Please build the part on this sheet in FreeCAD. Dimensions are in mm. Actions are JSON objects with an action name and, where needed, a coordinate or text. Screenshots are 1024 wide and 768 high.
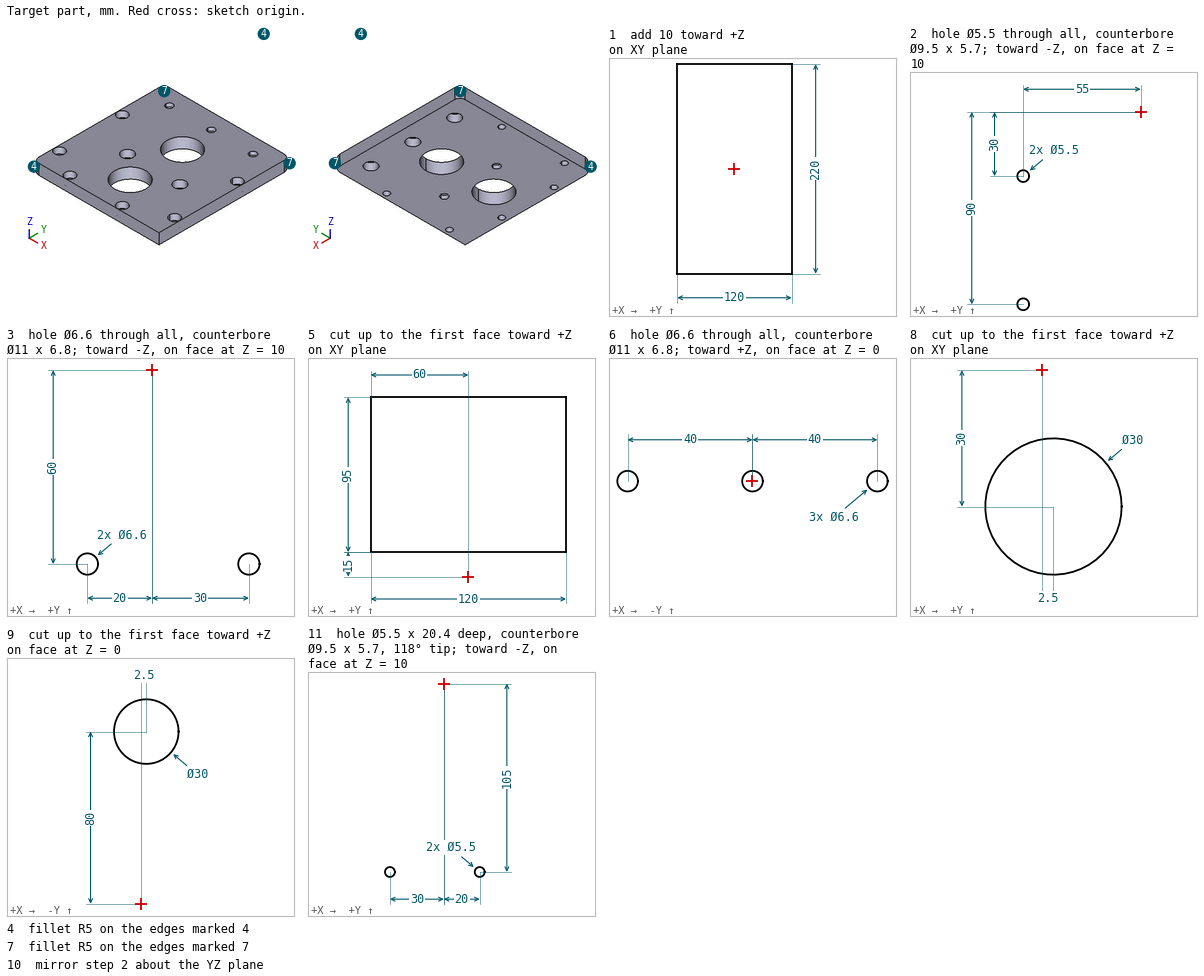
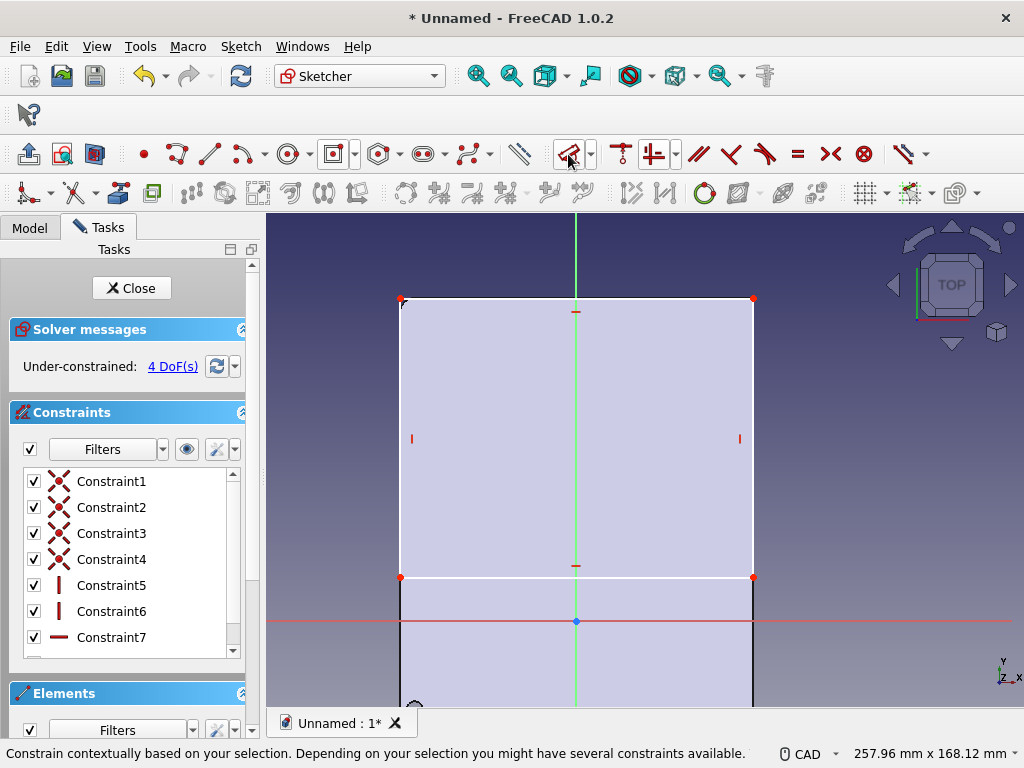
{"action": "left_click", "coordinate": [400, 383]}
{"action": "left_click", "coordinate": [366, 438]}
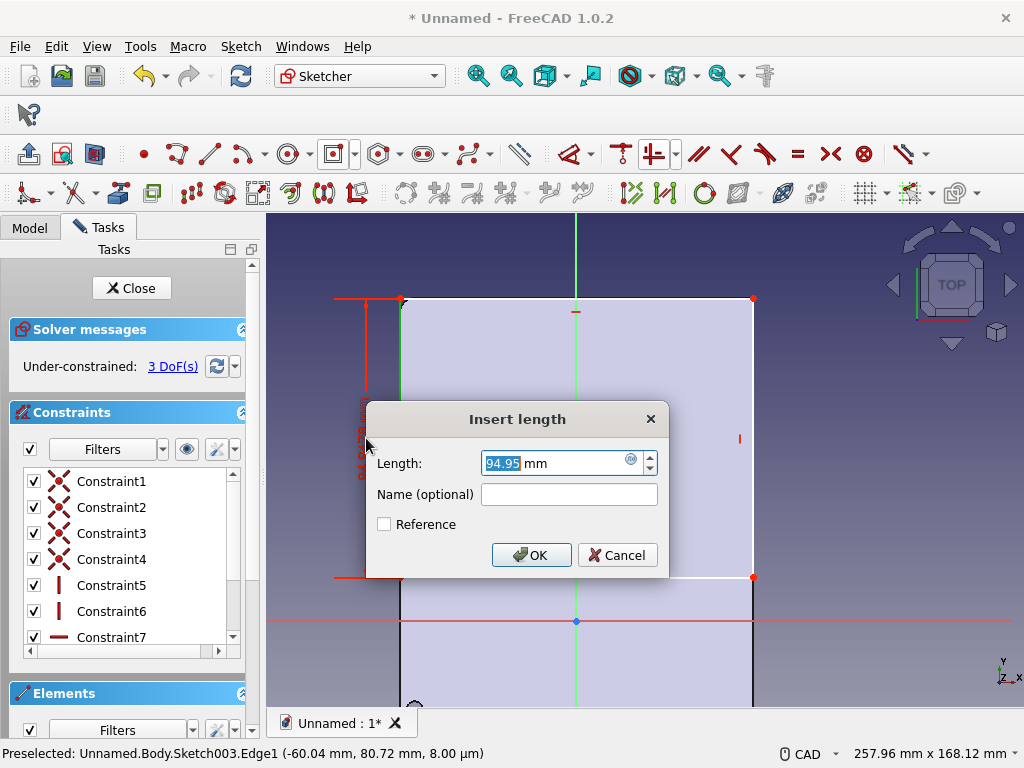
{"action": "type", "text": "95"}
{"action": "key", "text": "Return"}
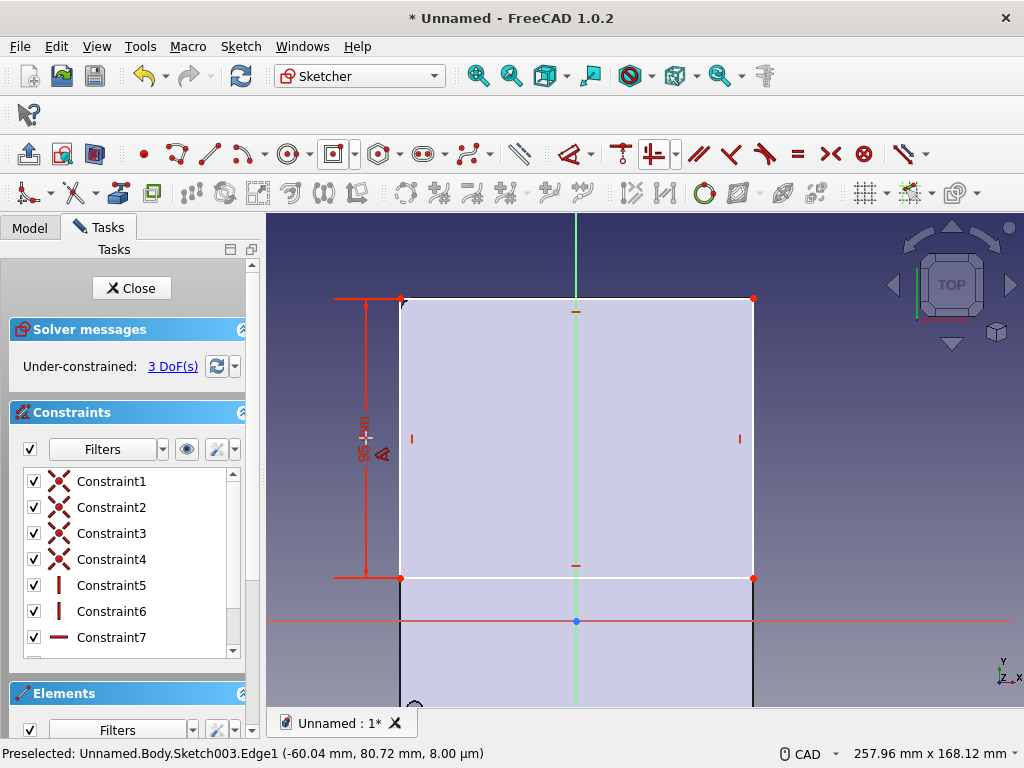
{"action": "left_click", "coordinate": [506, 578]}
{"action": "left_click", "coordinate": [495, 544]}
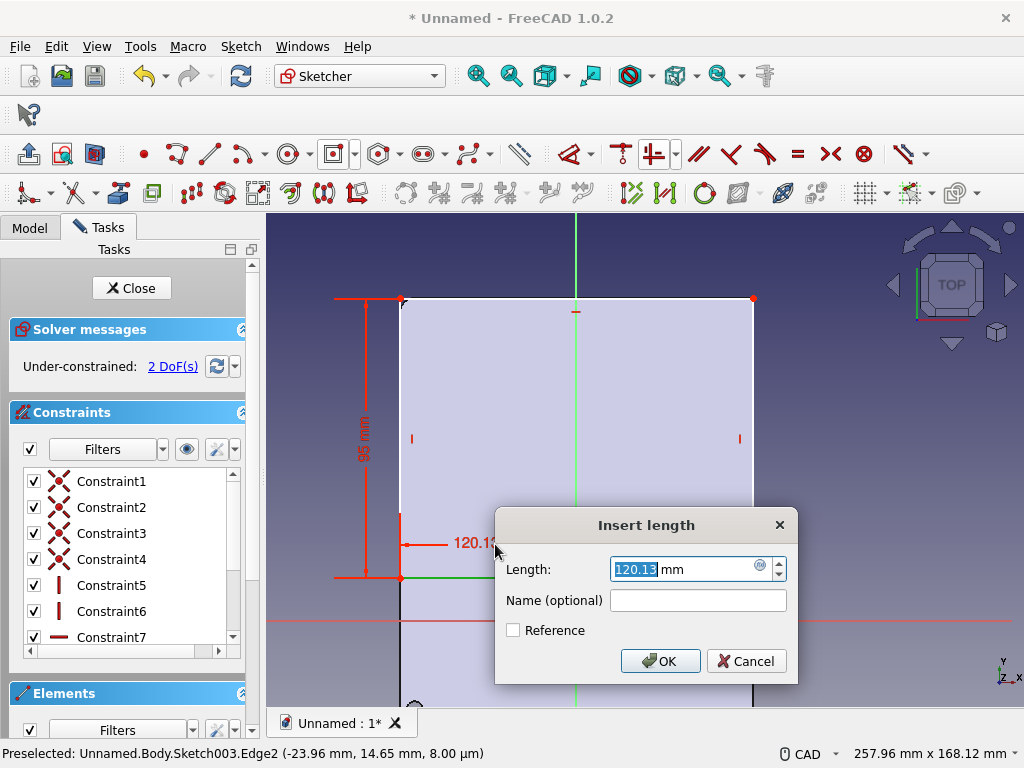
{"action": "type", "text": "120"}
{"action": "key", "text": "Return"}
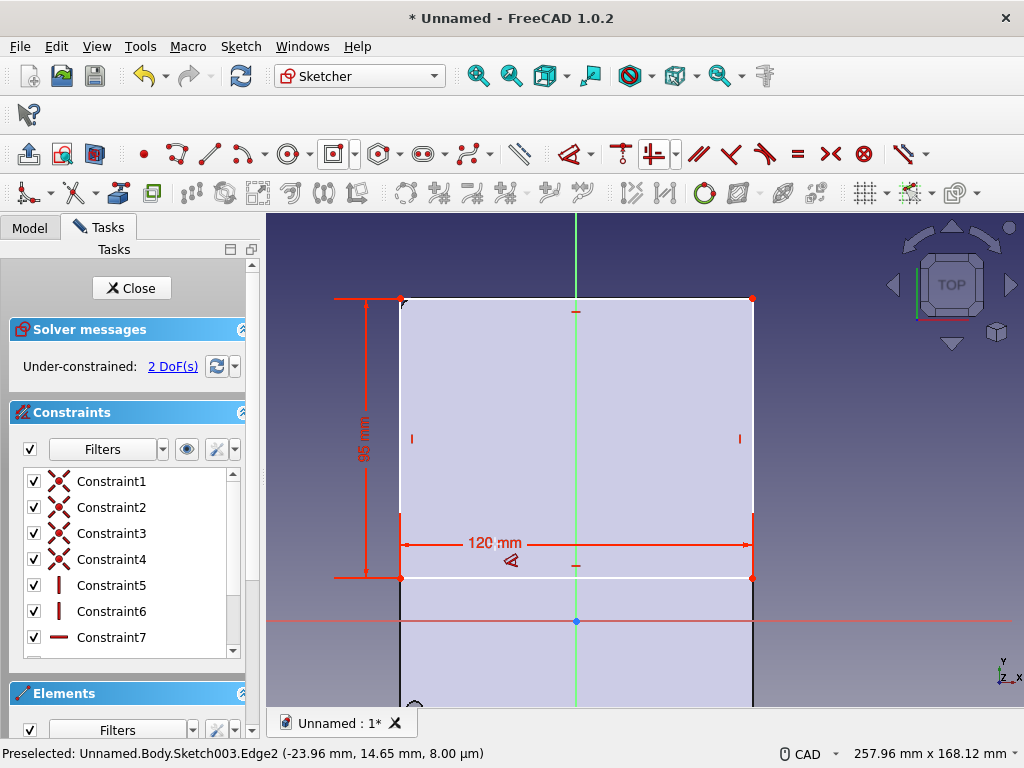
{"action": "left_click", "coordinate": [400, 299]}
{"action": "left_click", "coordinate": [488, 655]}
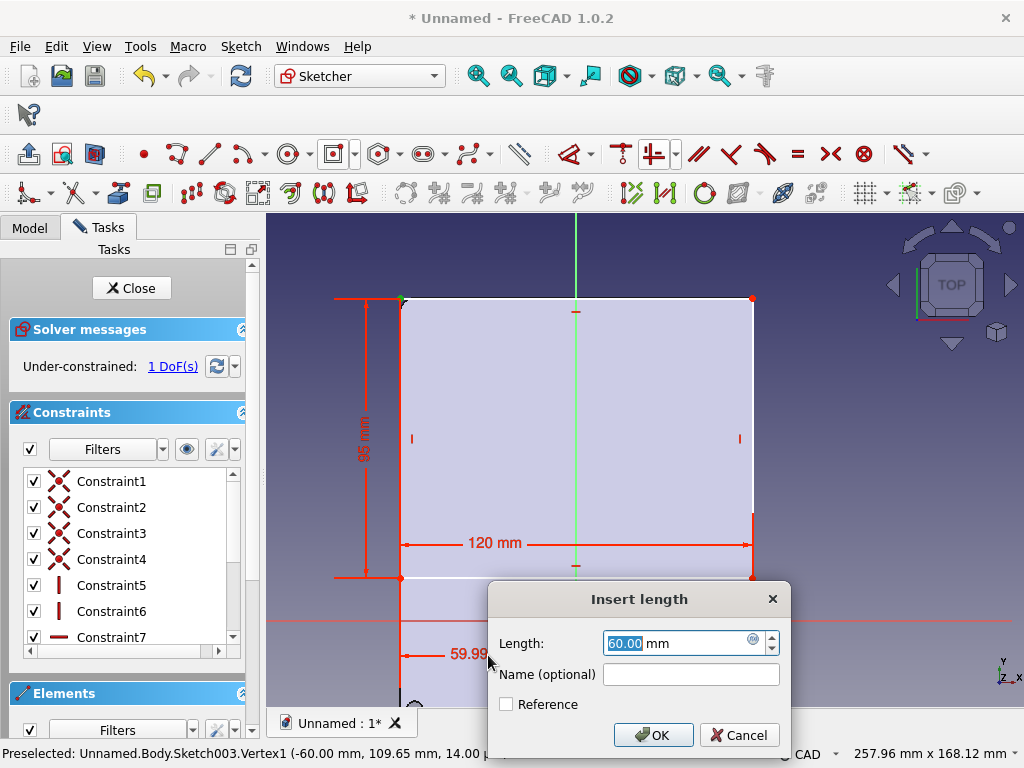
{"action": "type", "text": "60"}
{"action": "key", "text": "Return"}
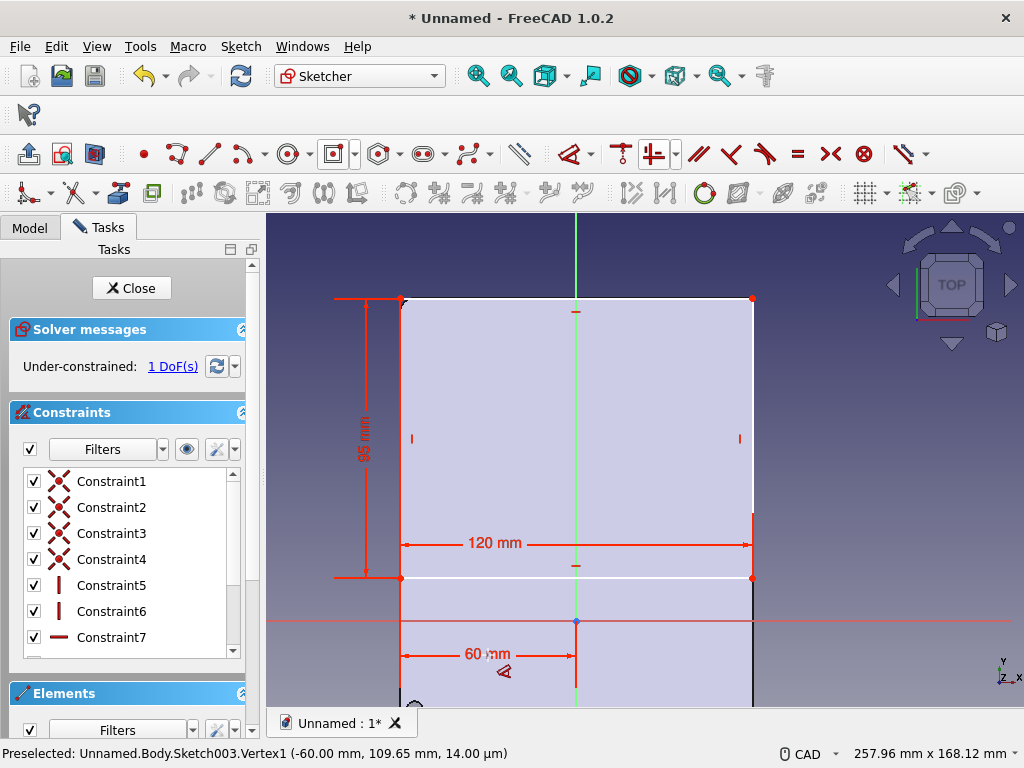
{"action": "left_click", "coordinate": [400, 578]}
{"action": "left_click", "coordinate": [366, 600]}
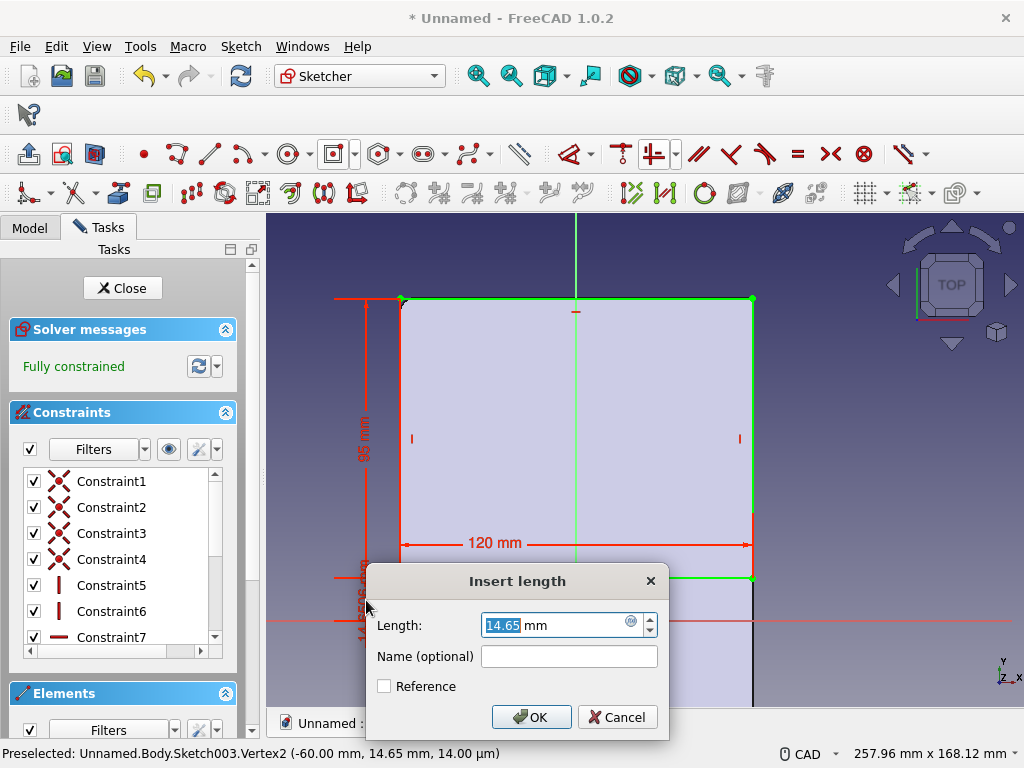
{"action": "type", "text": "15"}
{"action": "key", "text": "Return"}
{"action": "key", "text": "Escape"}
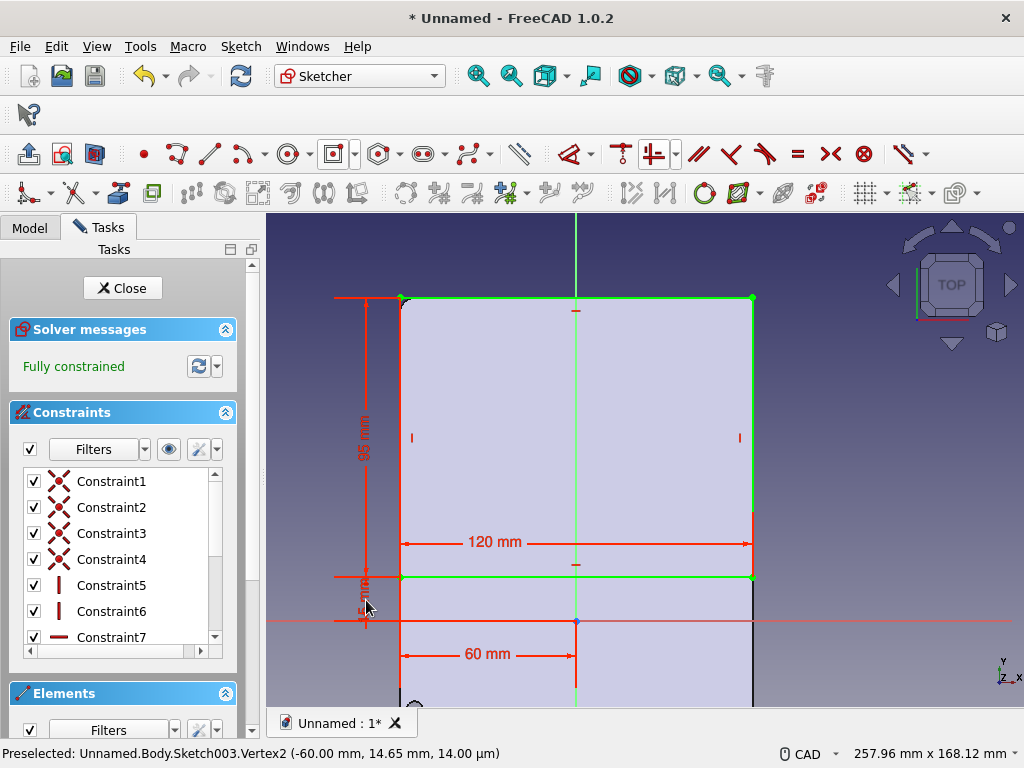
{"action": "left_click", "coordinate": [123, 288]}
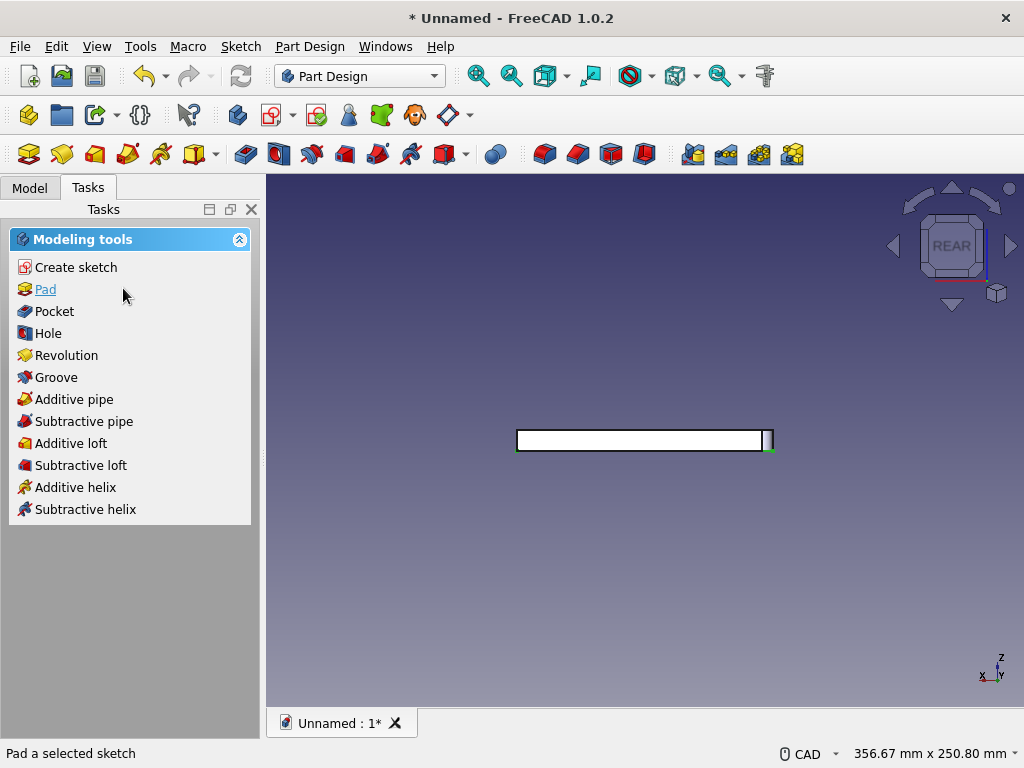
{"action": "left_click", "coordinate": [246, 154]}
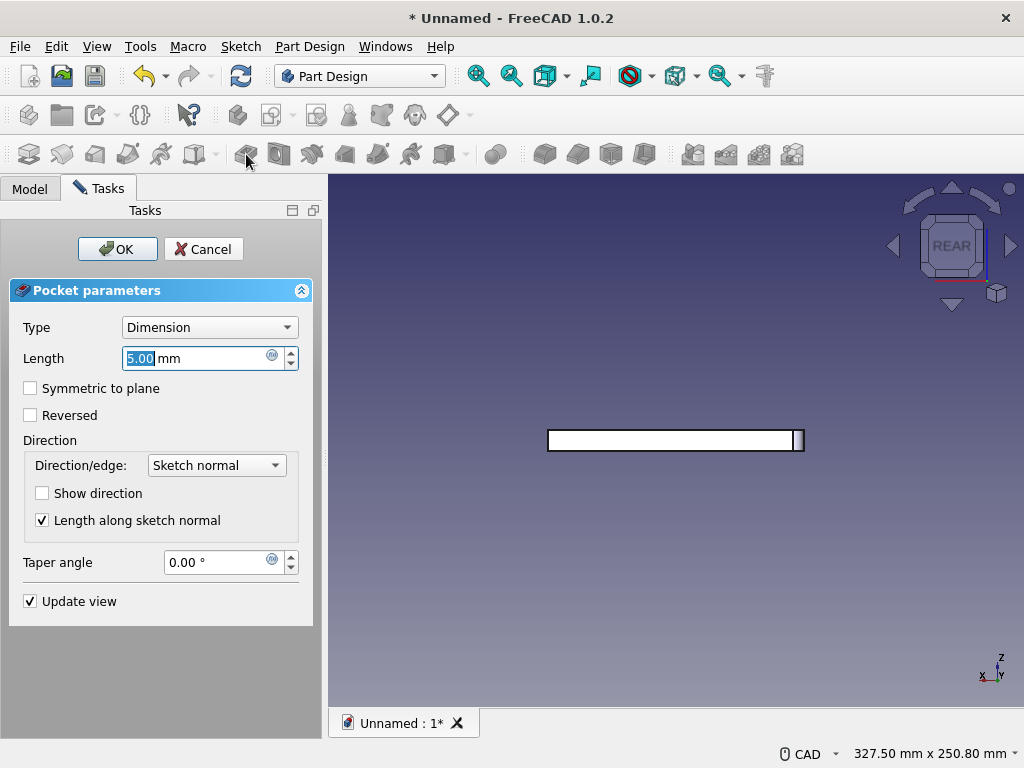
{"action": "left_click", "coordinate": [210, 328]}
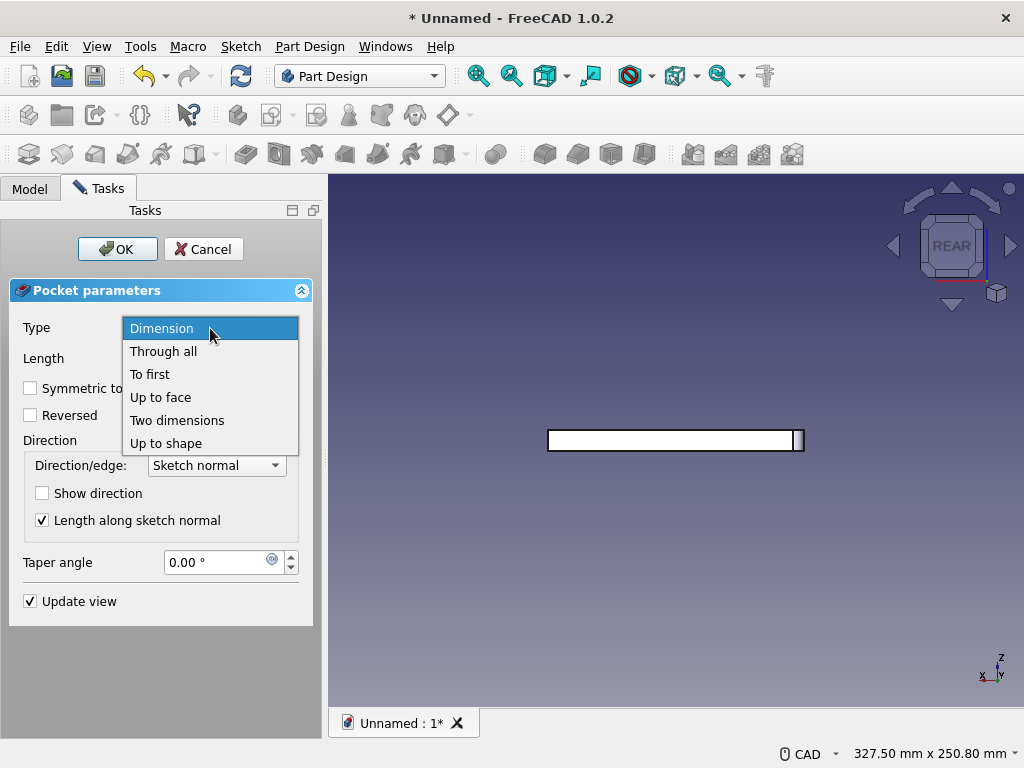
{"action": "left_click", "coordinate": [208, 374]}